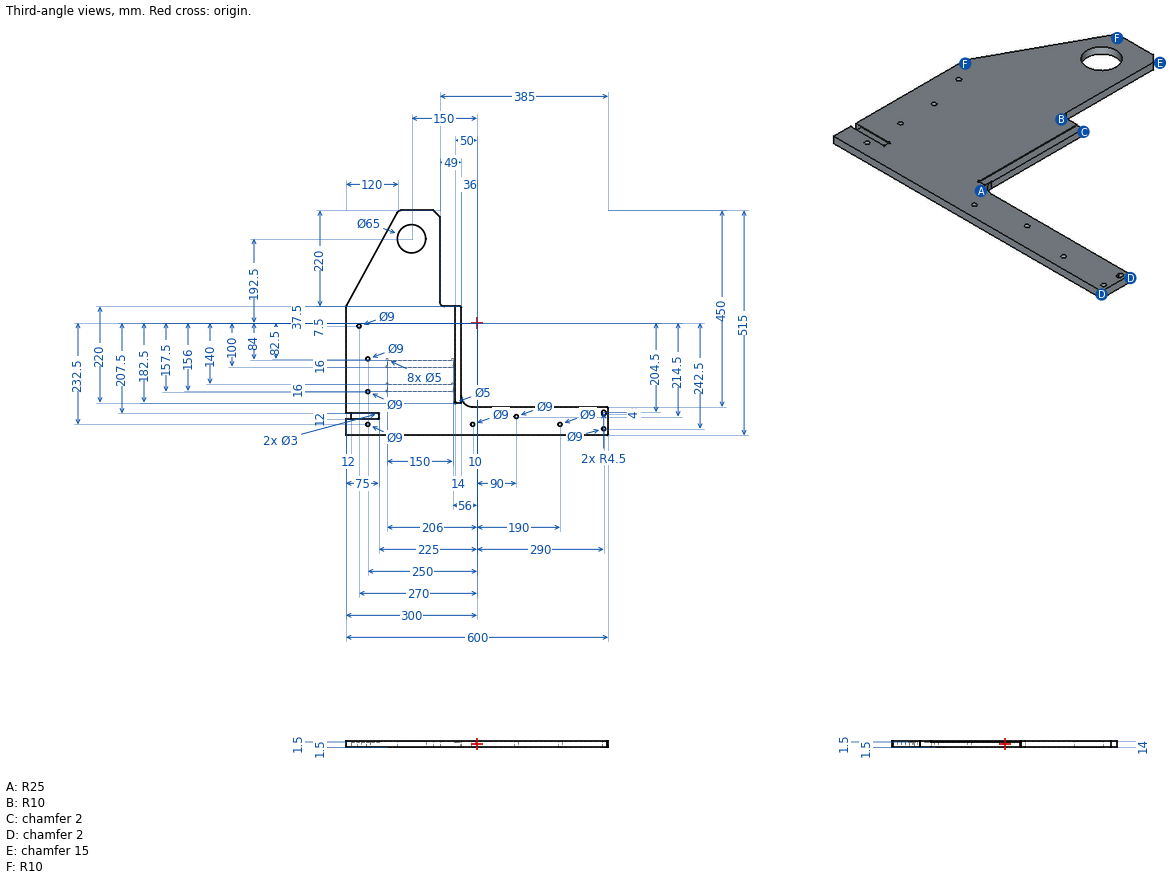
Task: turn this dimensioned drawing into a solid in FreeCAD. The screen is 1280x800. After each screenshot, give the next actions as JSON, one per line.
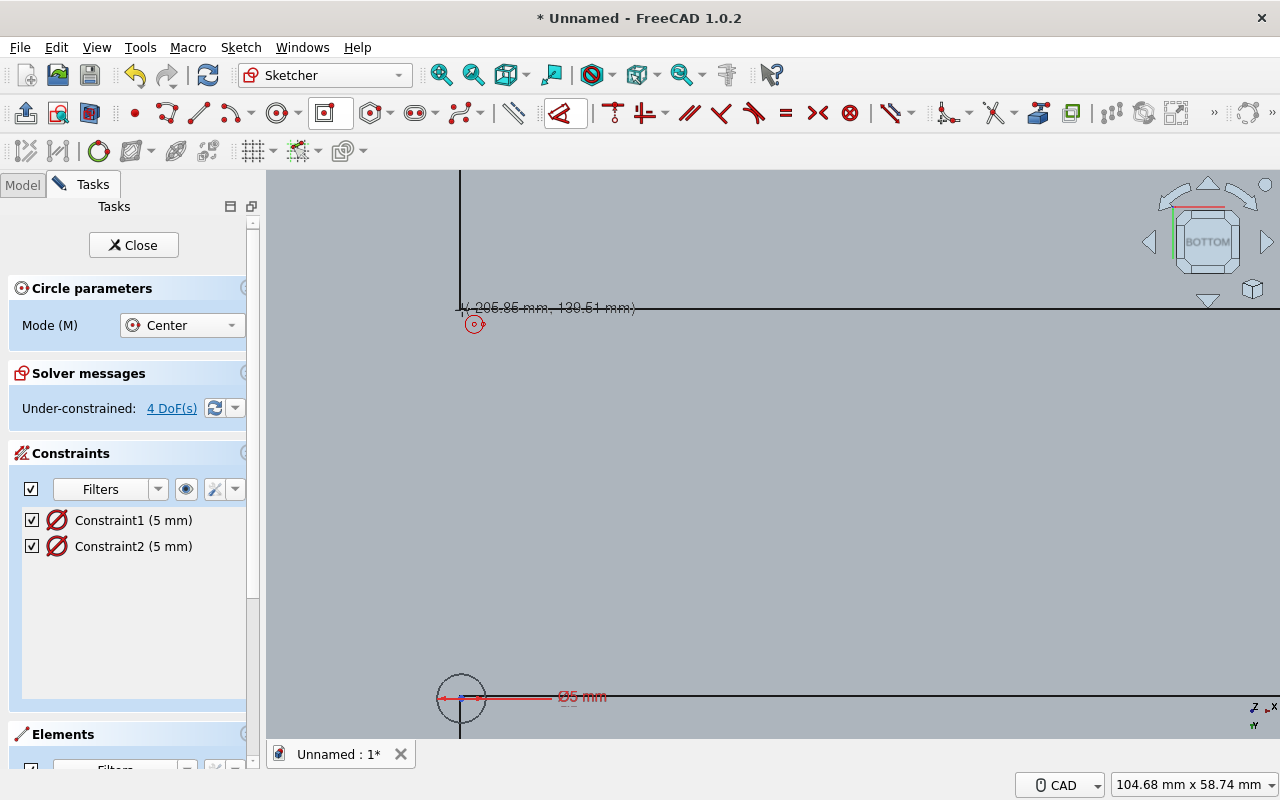
{"action": "scroll", "coordinate": [462, 310], "scroll_direction": "down", "scroll_amount": 7}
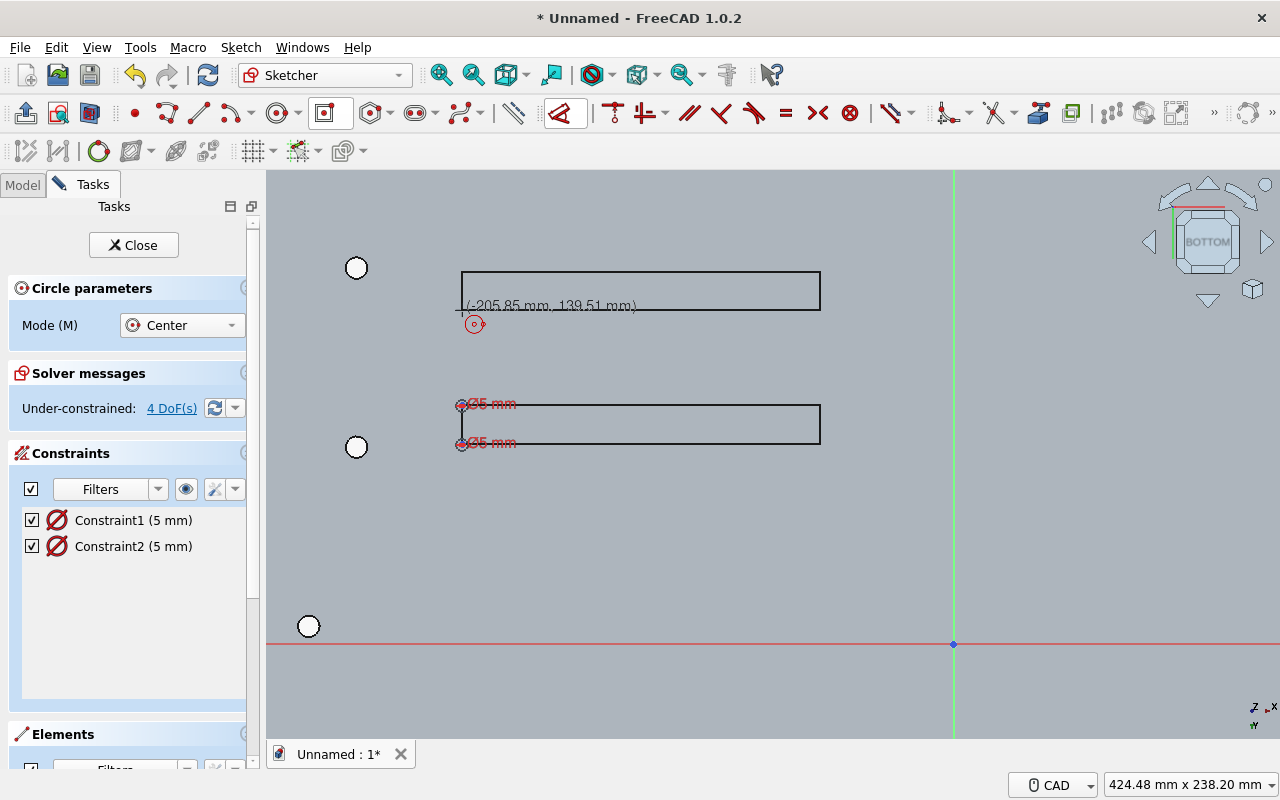
{"action": "left_click", "coordinate": [462, 310]}
{"action": "mouse_move", "coordinate": [466, 306]}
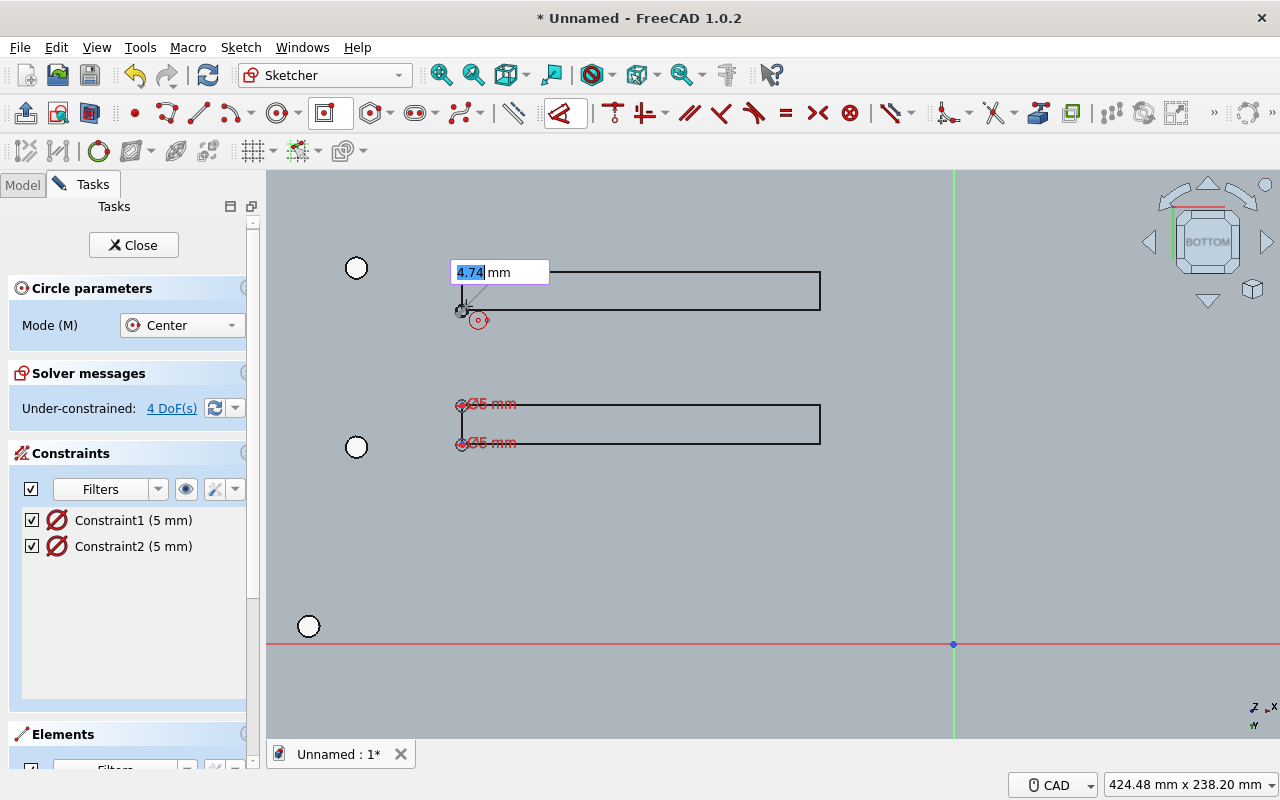
{"action": "type", "text": "5"}
{"action": "key", "text": "Return"}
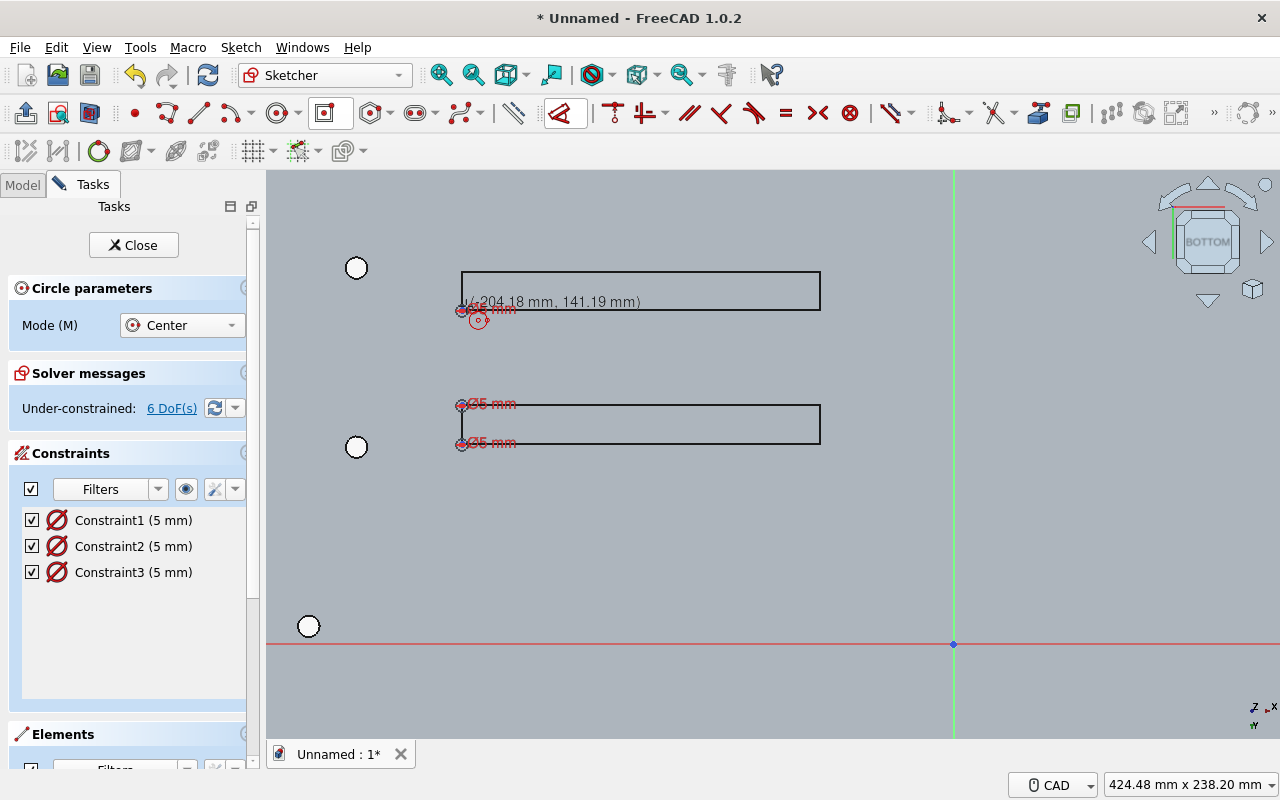
{"action": "scroll", "coordinate": [462, 272], "scroll_direction": "up", "scroll_amount": 7}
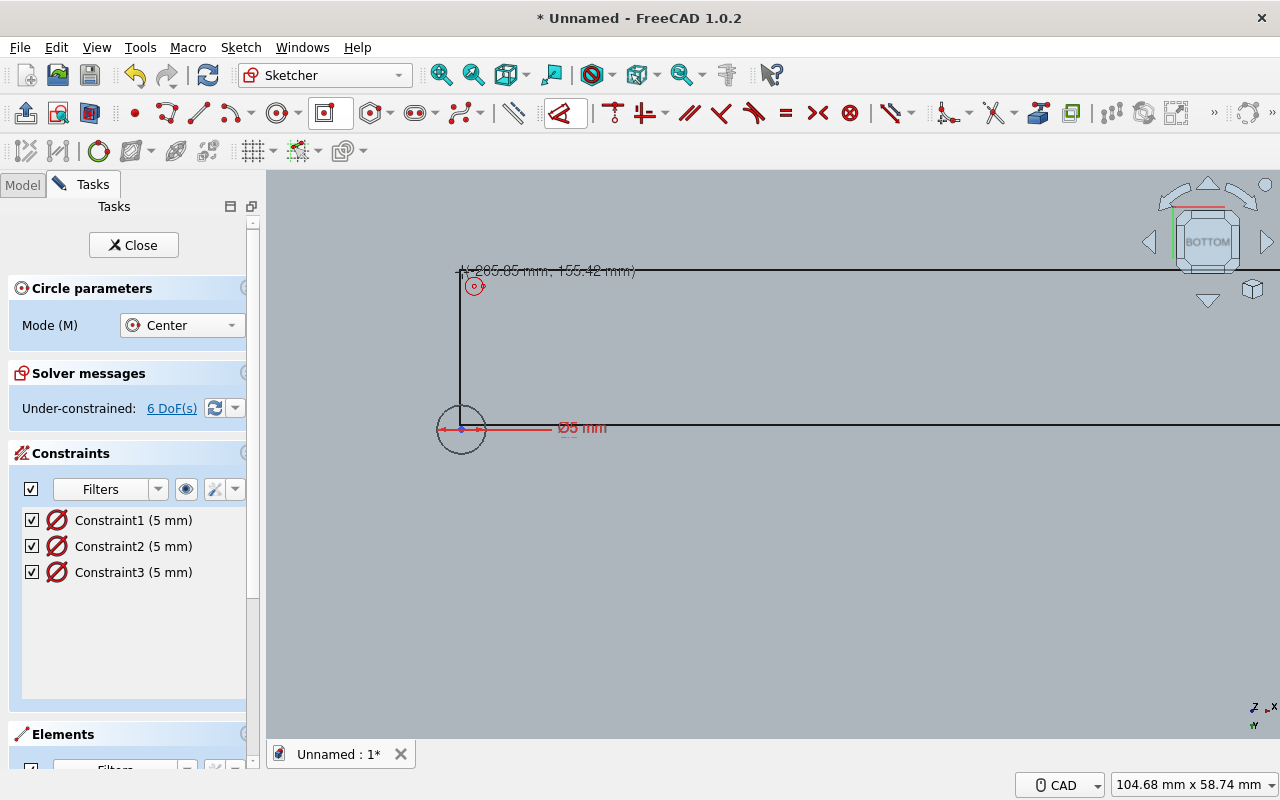
{"action": "scroll", "coordinate": [462, 272], "scroll_direction": "down", "scroll_amount": 7}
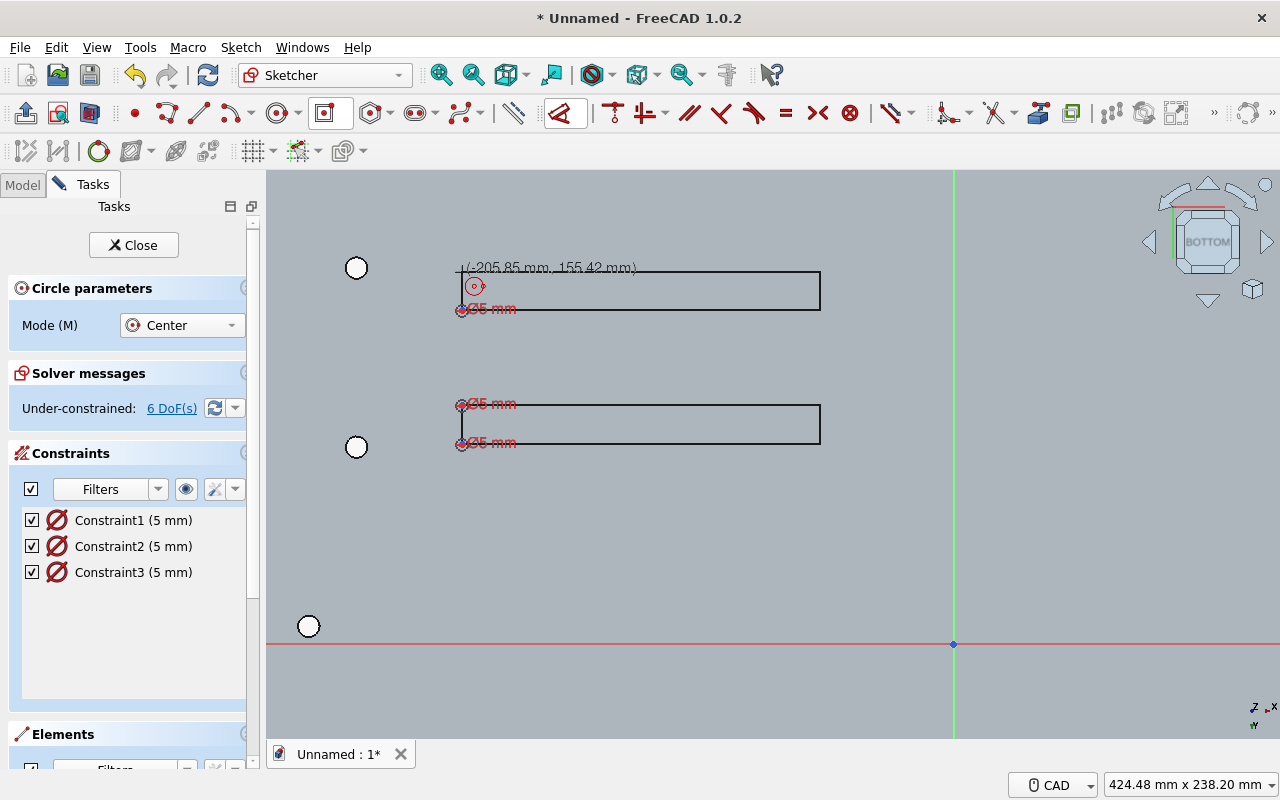
{"action": "left_click", "coordinate": [462, 272]}
{"action": "mouse_move", "coordinate": [466, 267]}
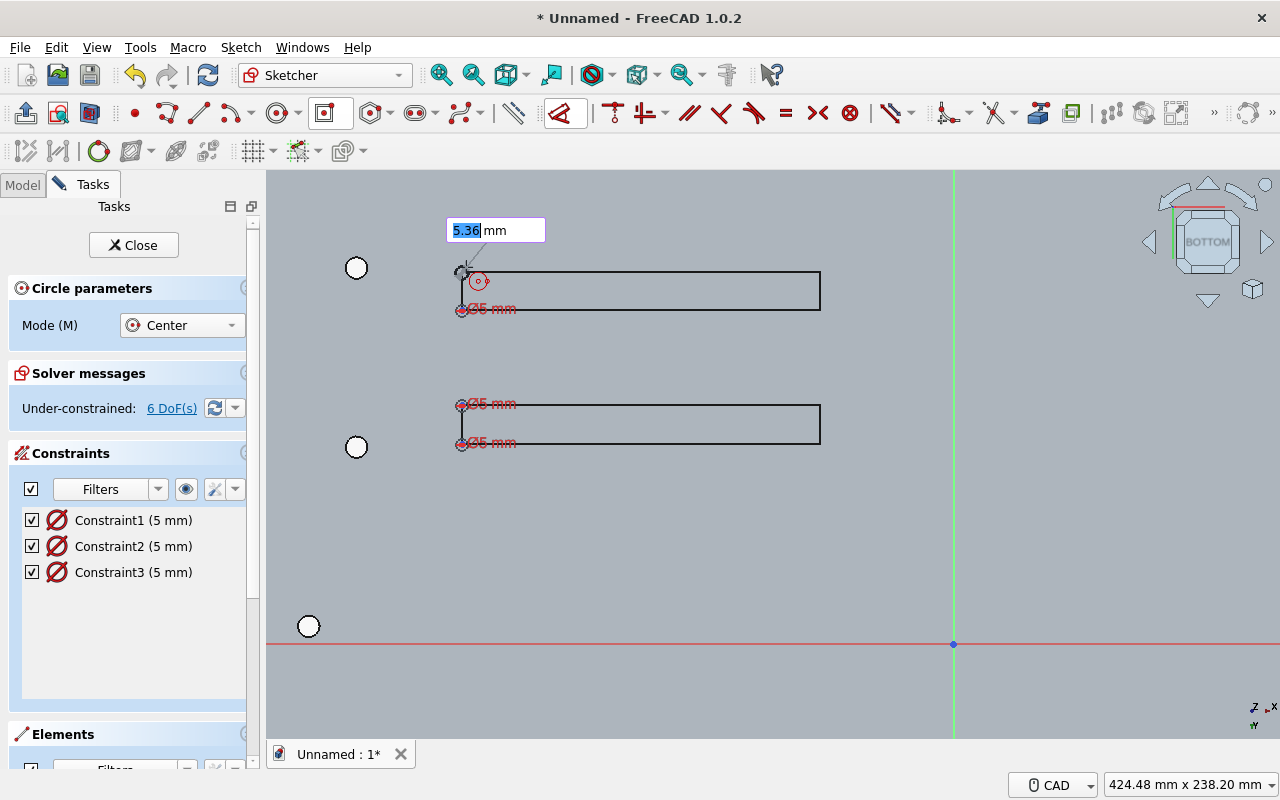
{"action": "type", "text": "5"}
{"action": "key", "text": "Return"}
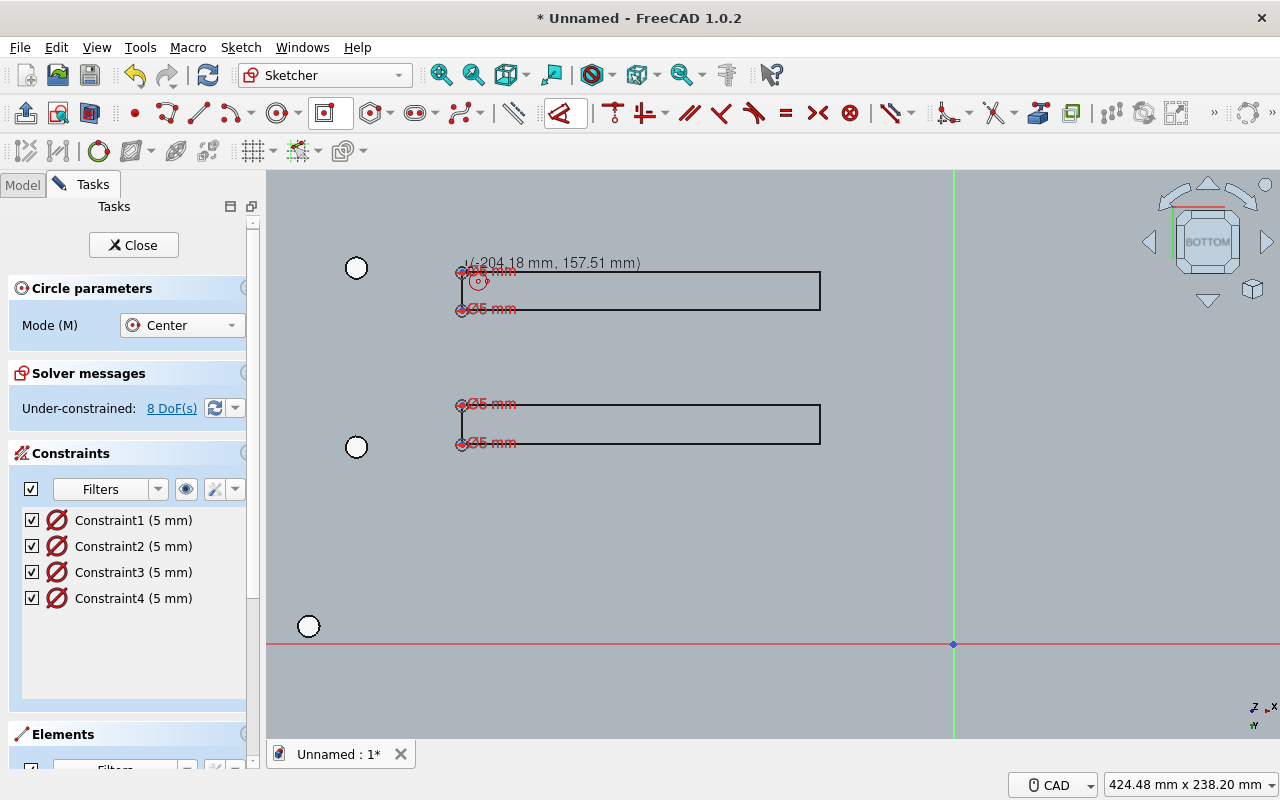
{"action": "scroll", "coordinate": [820, 444], "scroll_direction": "up", "scroll_amount": 7}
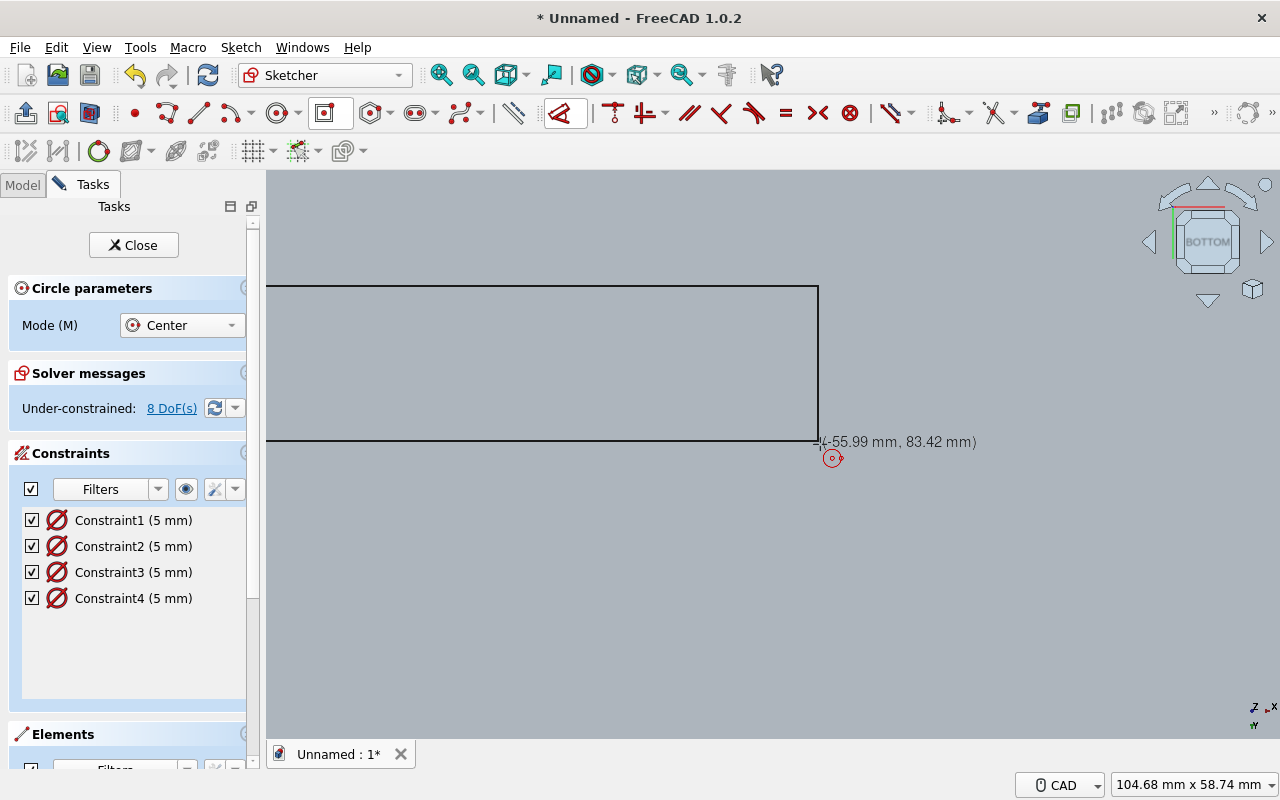
{"action": "scroll", "coordinate": [820, 444], "scroll_direction": "down", "scroll_amount": 7}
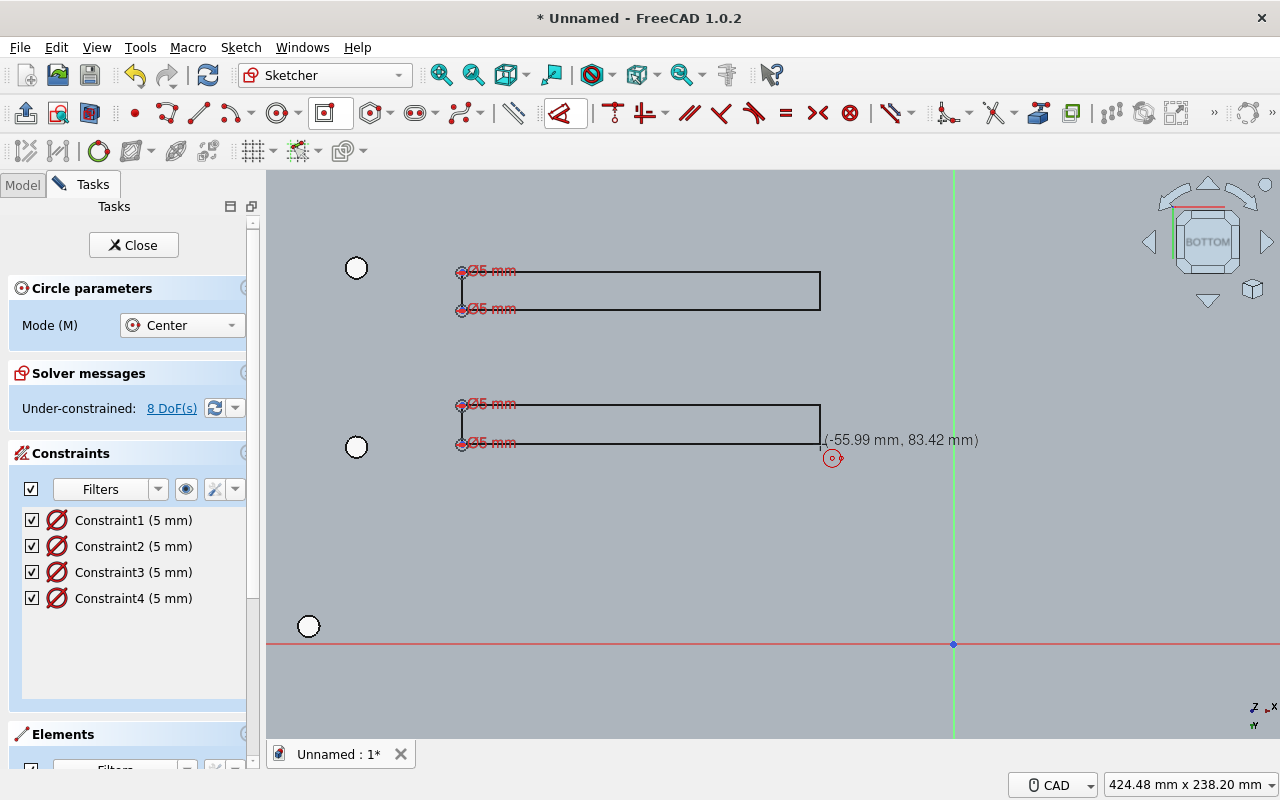
{"action": "left_click", "coordinate": [820, 444]}
{"action": "mouse_move", "coordinate": [824, 439]}